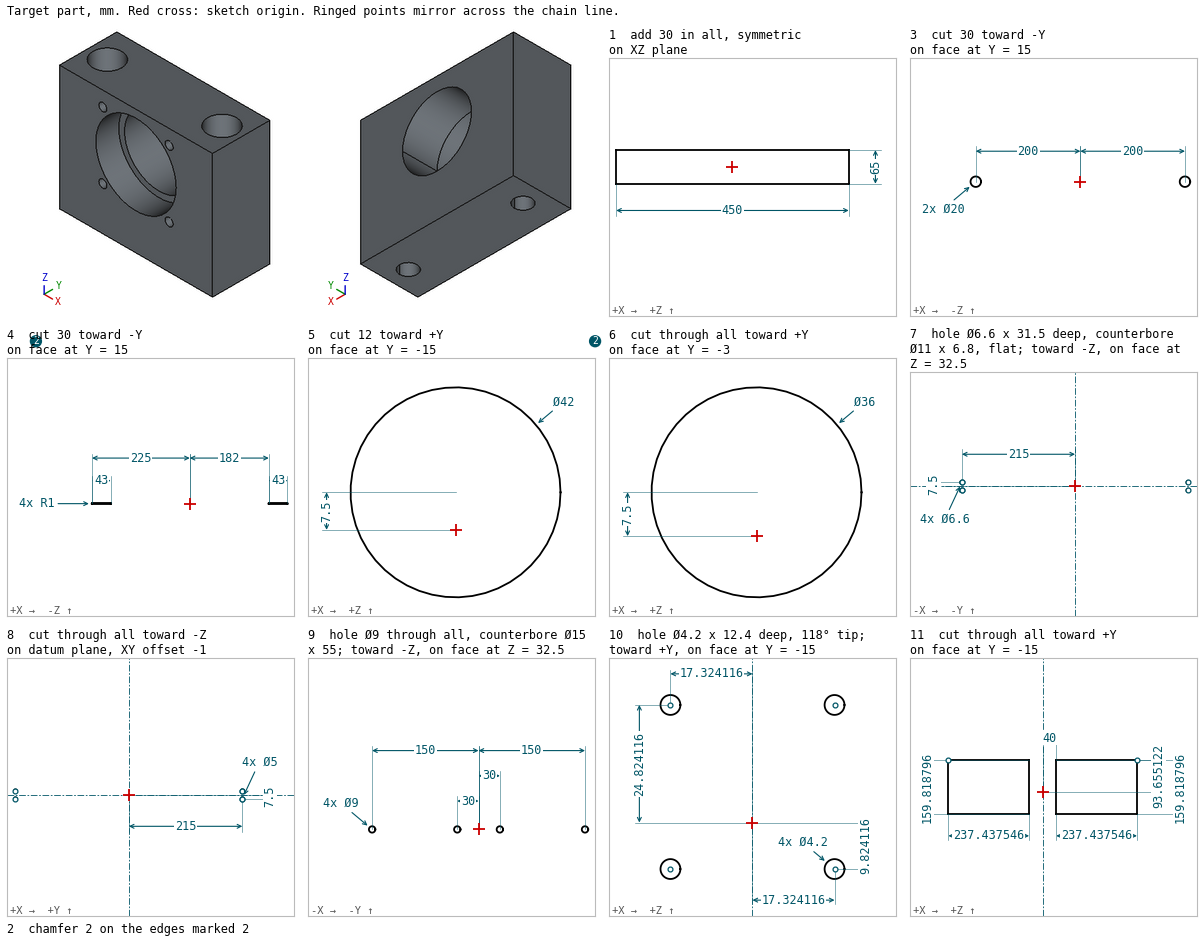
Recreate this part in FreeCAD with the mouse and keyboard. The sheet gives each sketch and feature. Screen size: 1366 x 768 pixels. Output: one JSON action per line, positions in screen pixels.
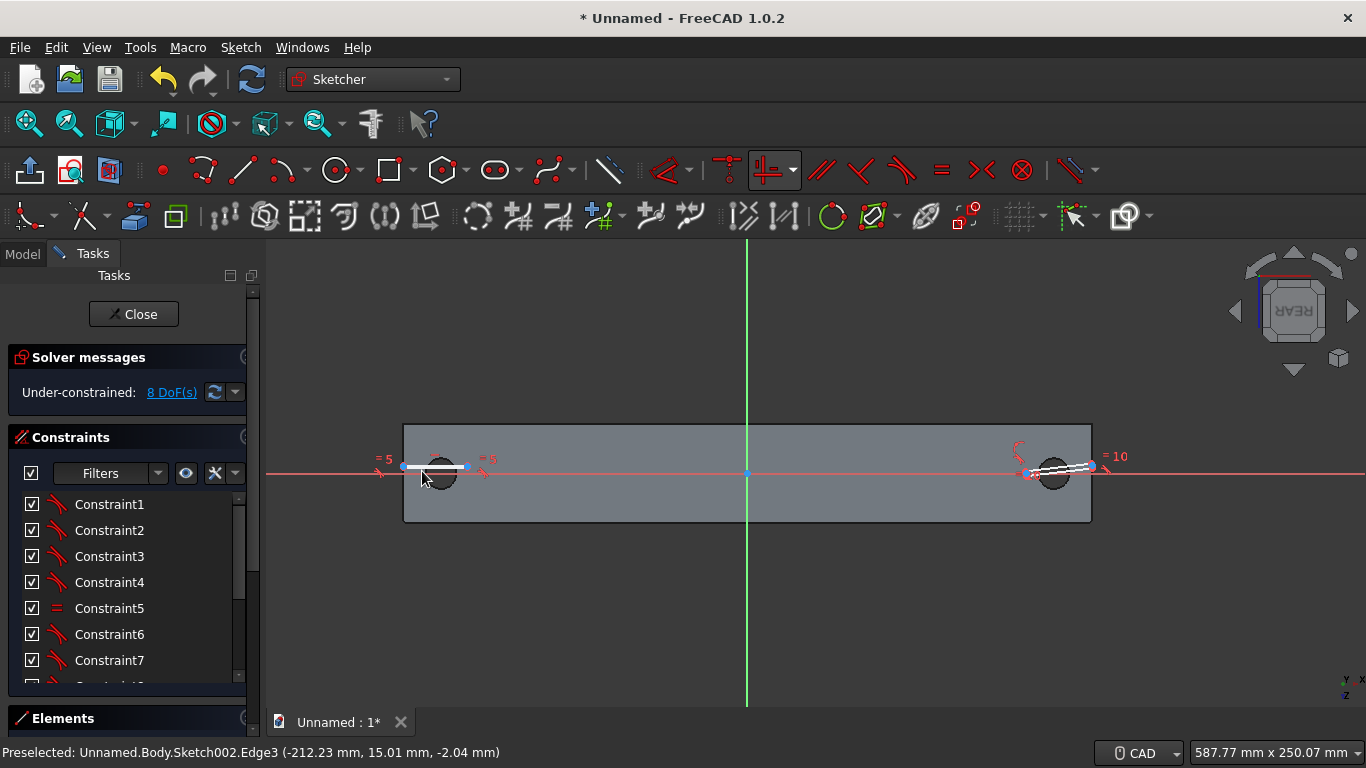
{"action": "scroll", "coordinate": [1046, 469], "scroll_direction": "up", "scroll_amount": 6}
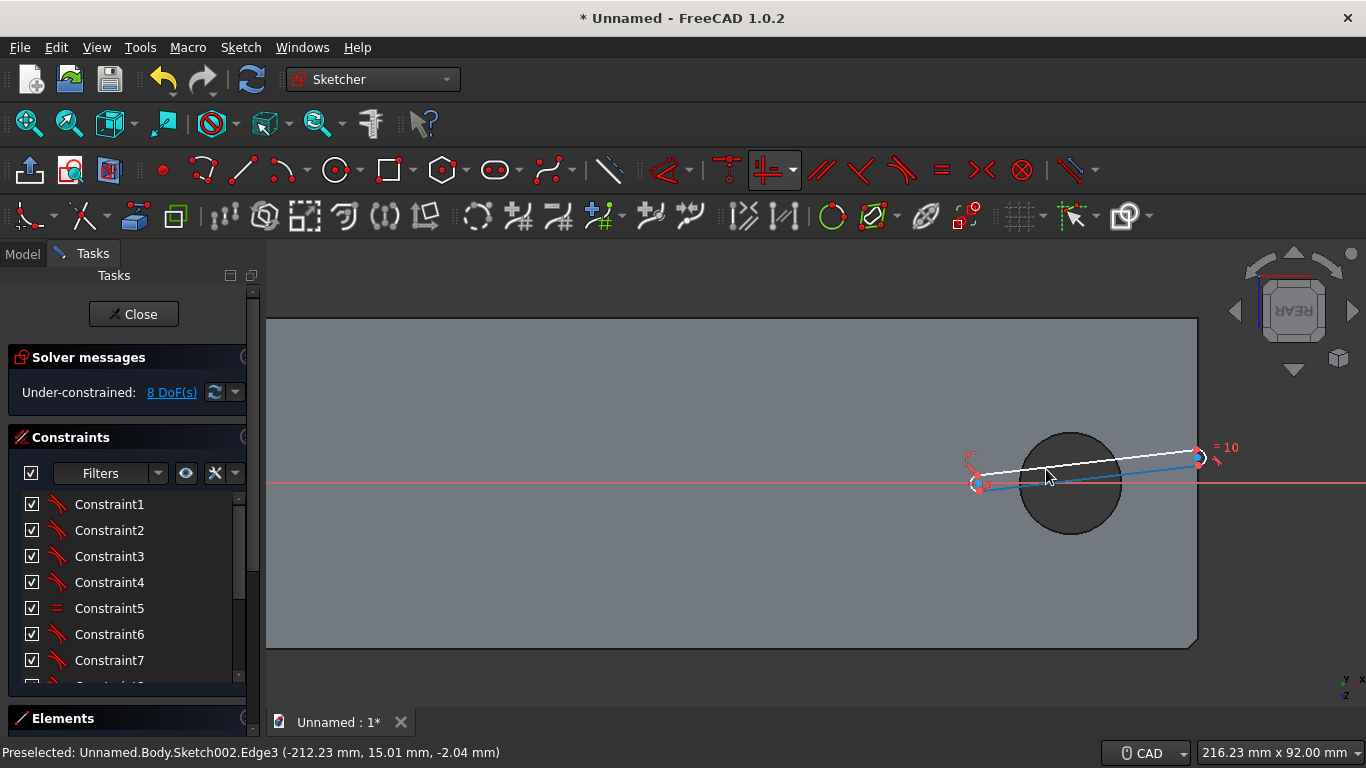
{"action": "left_click", "coordinate": [1043, 468]}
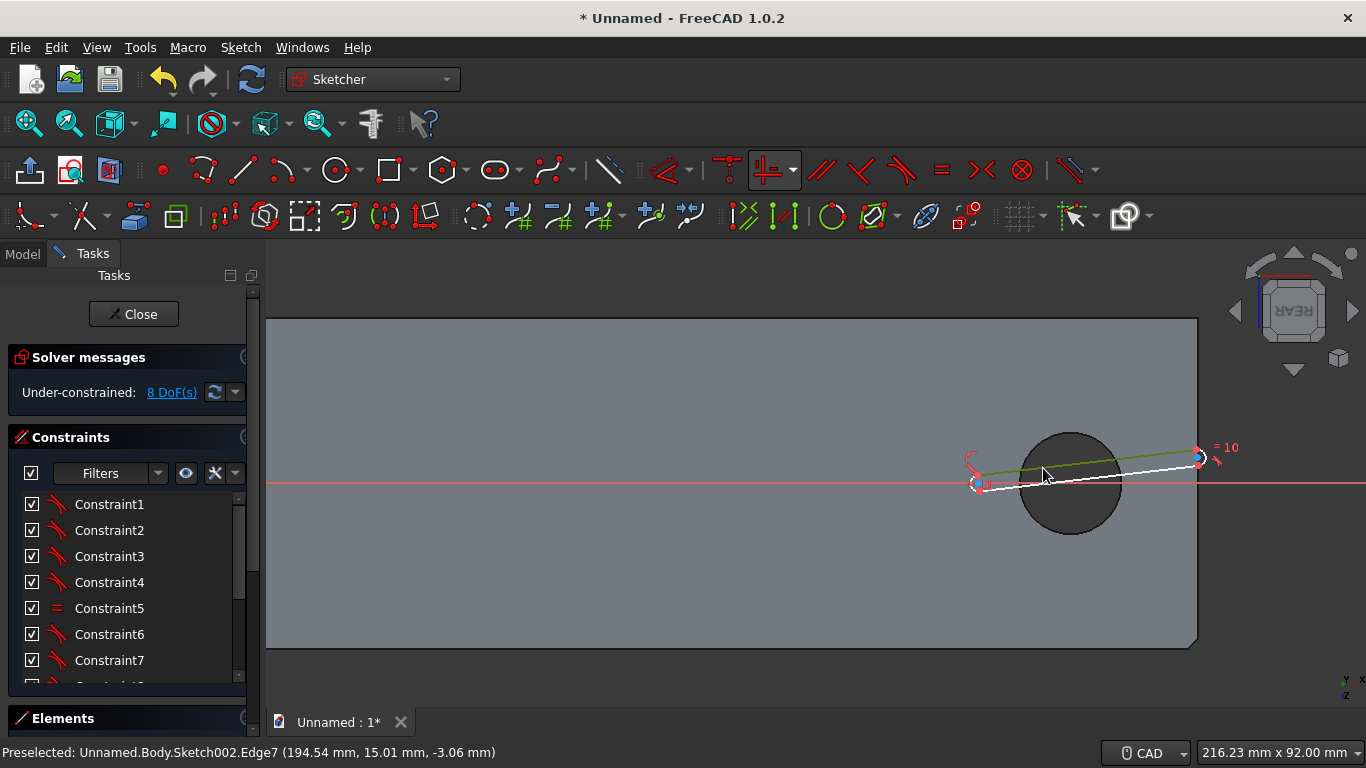
{"action": "key", "text": "h"}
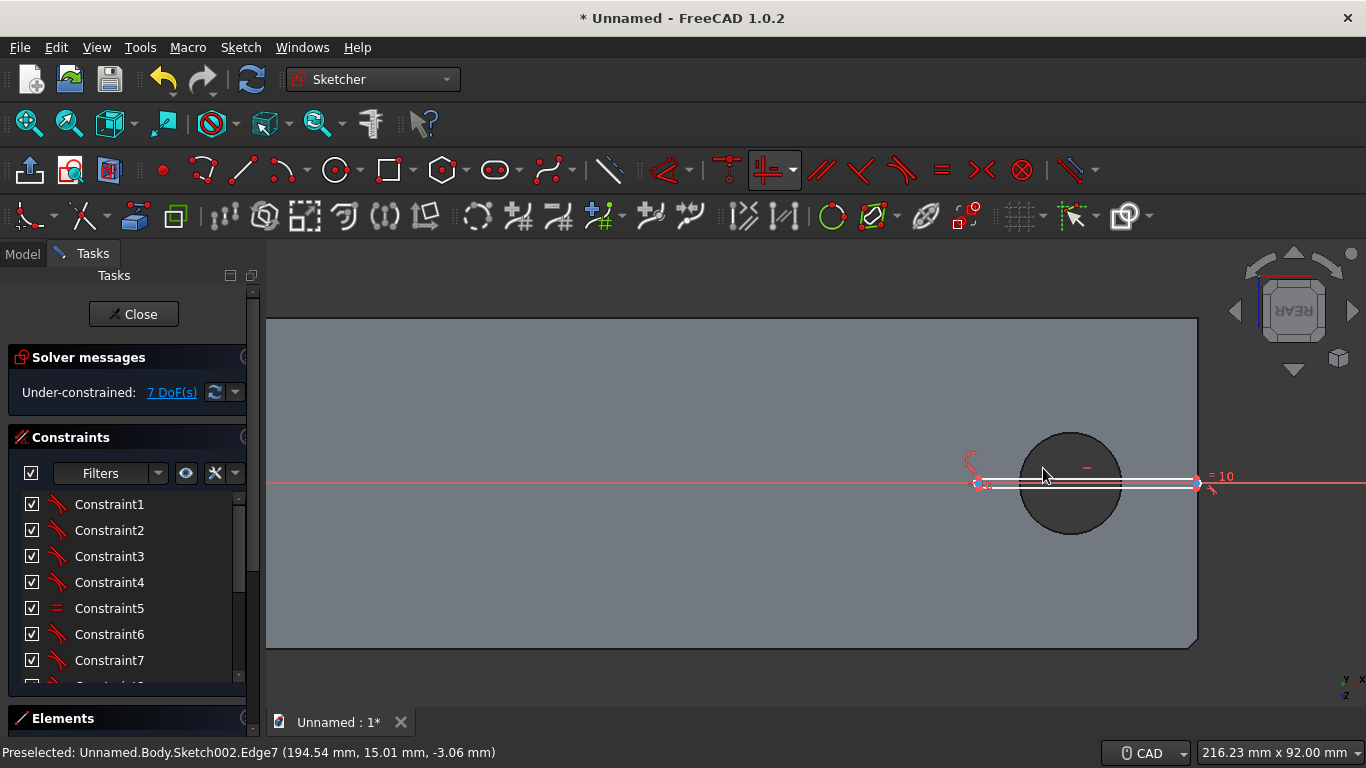
{"action": "scroll", "coordinate": [1047, 468], "scroll_direction": "down", "scroll_amount": 6}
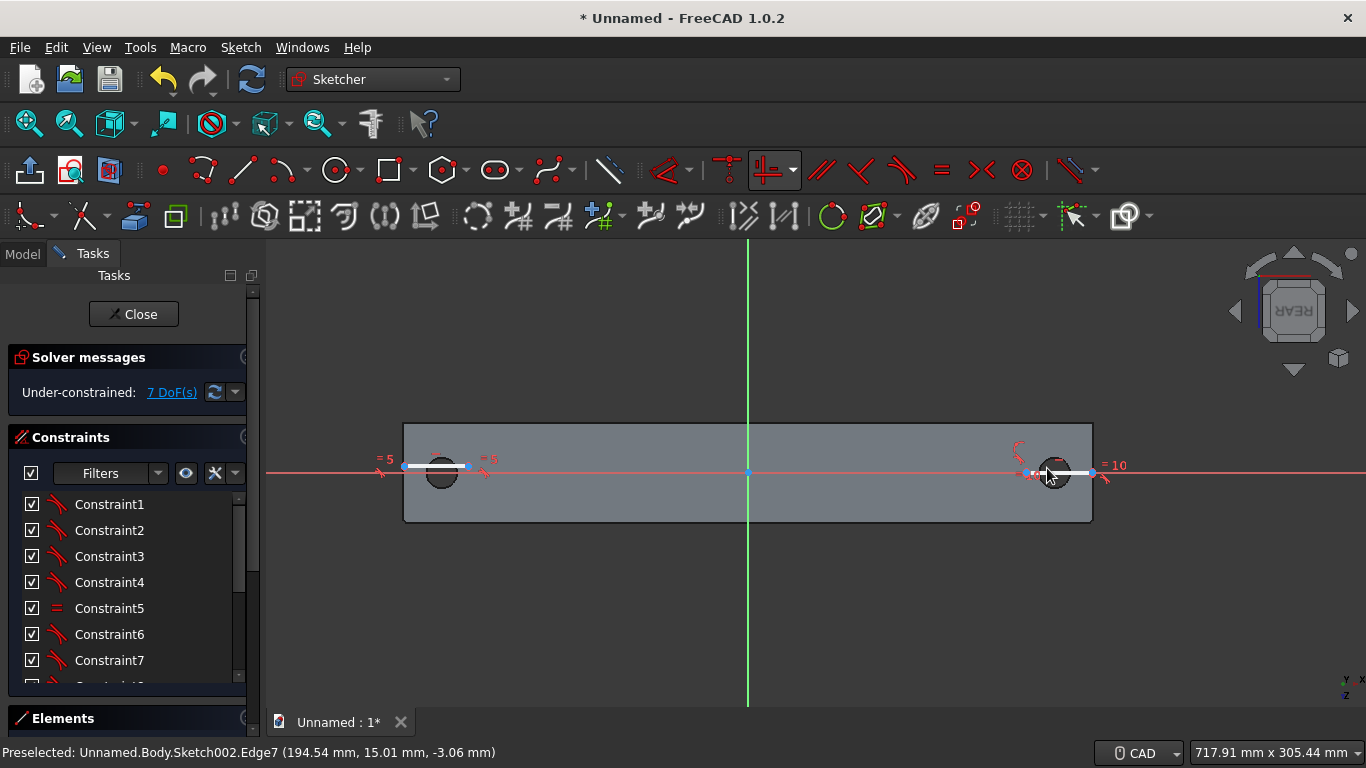
{"action": "scroll", "coordinate": [403, 466], "scroll_direction": "up", "scroll_amount": 13}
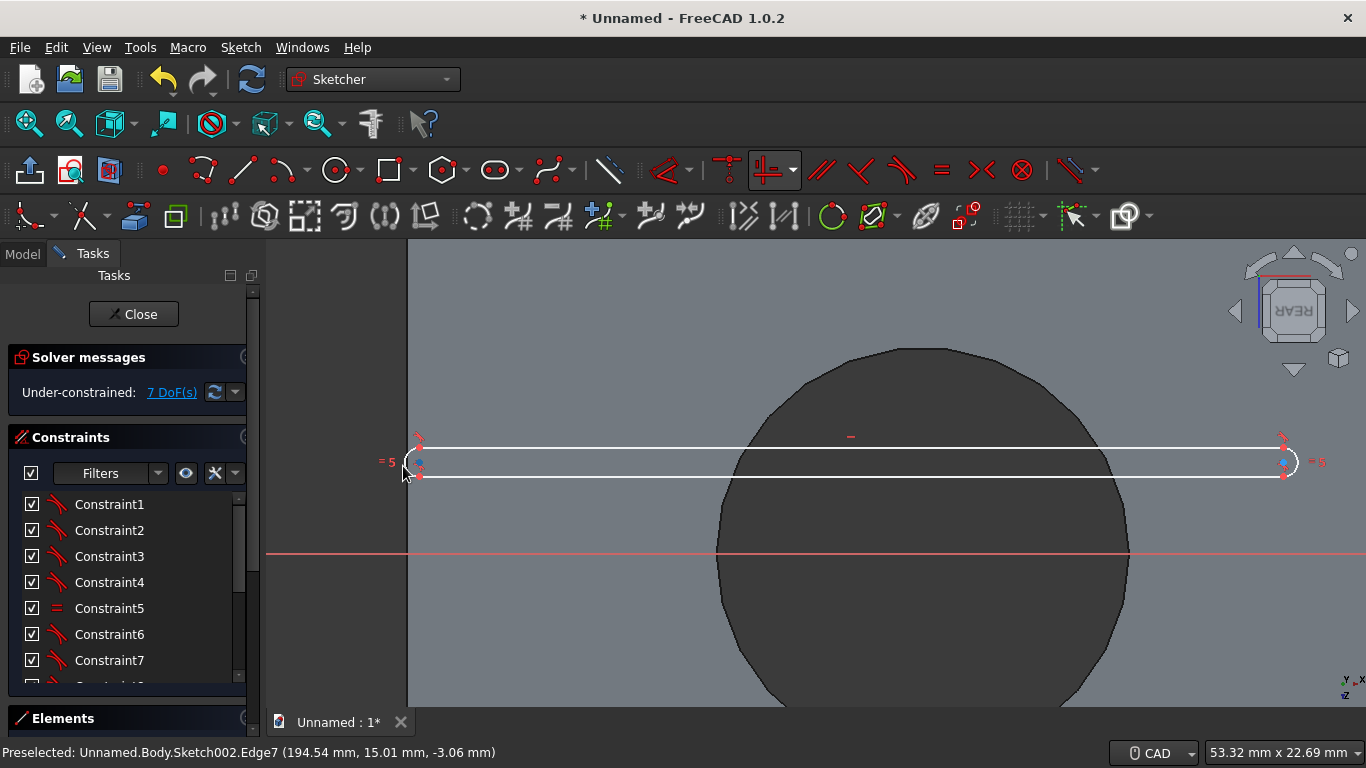
{"action": "left_click", "coordinate": [405, 462]}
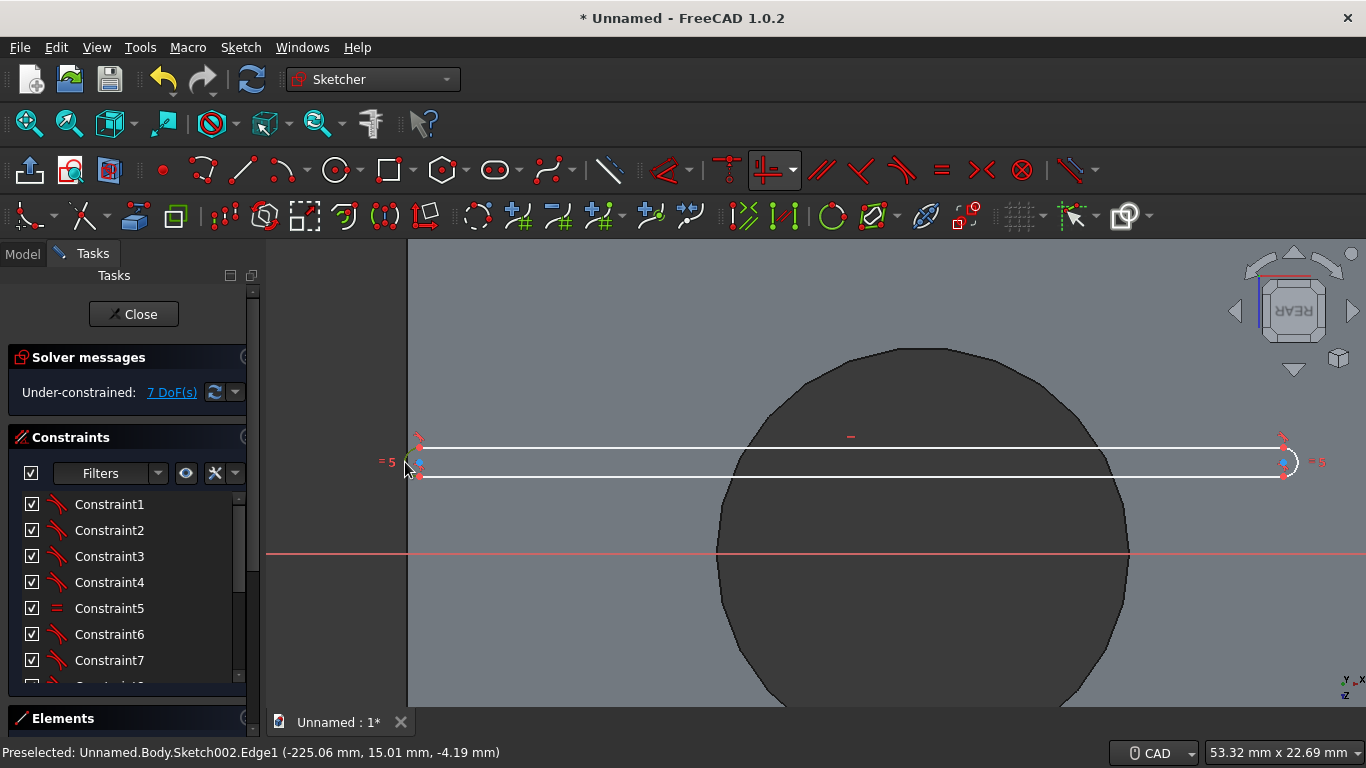
{"action": "scroll", "coordinate": [402, 466], "scroll_direction": "down", "scroll_amount": 13}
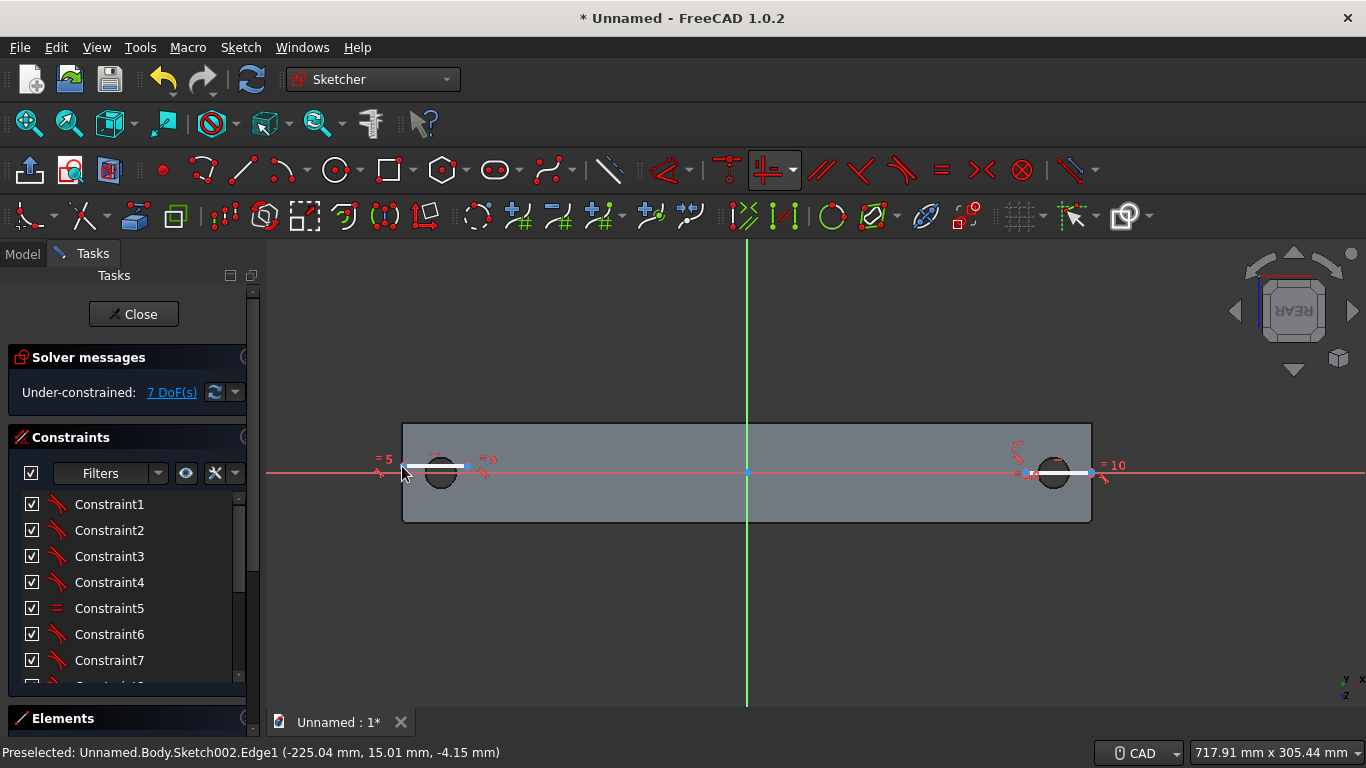
{"action": "scroll", "coordinate": [1025, 472], "scroll_direction": "up", "scroll_amount": 14}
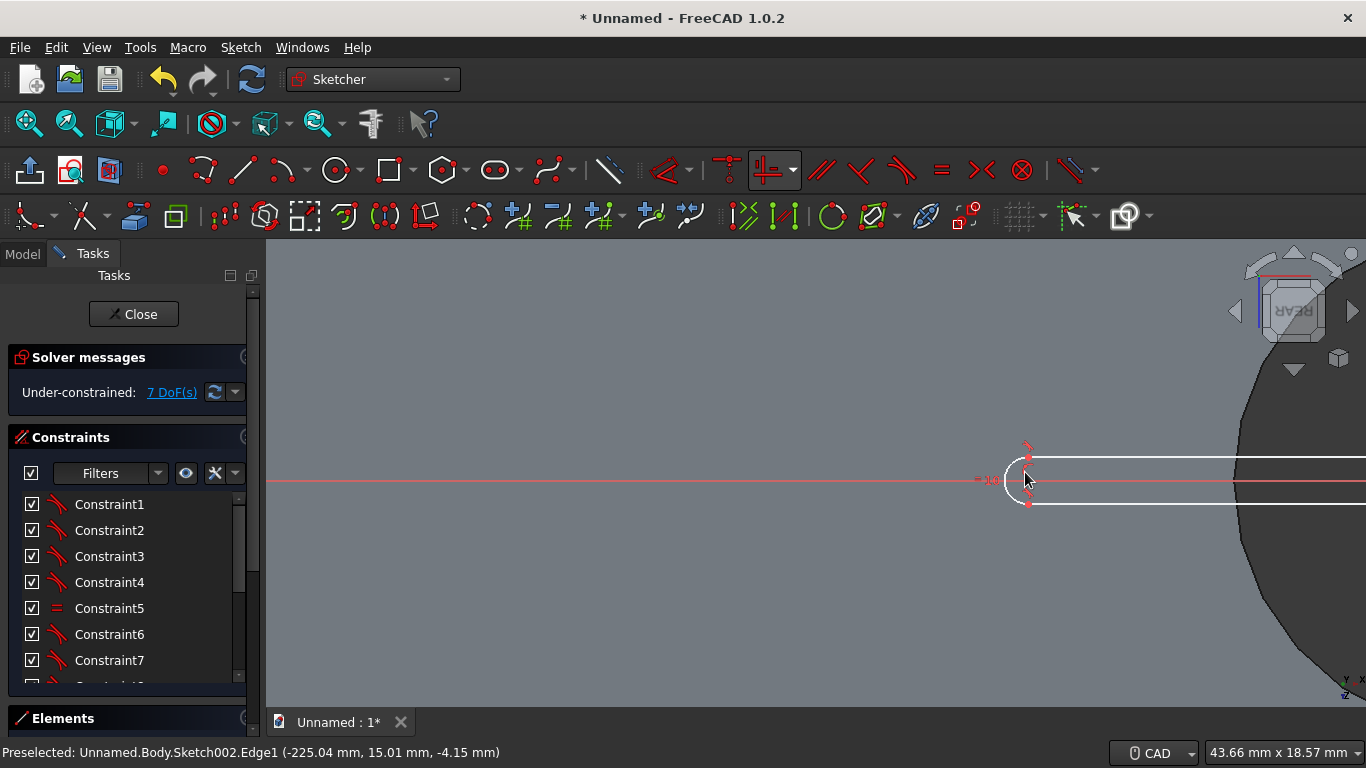
{"action": "left_click", "coordinate": [1009, 467]}